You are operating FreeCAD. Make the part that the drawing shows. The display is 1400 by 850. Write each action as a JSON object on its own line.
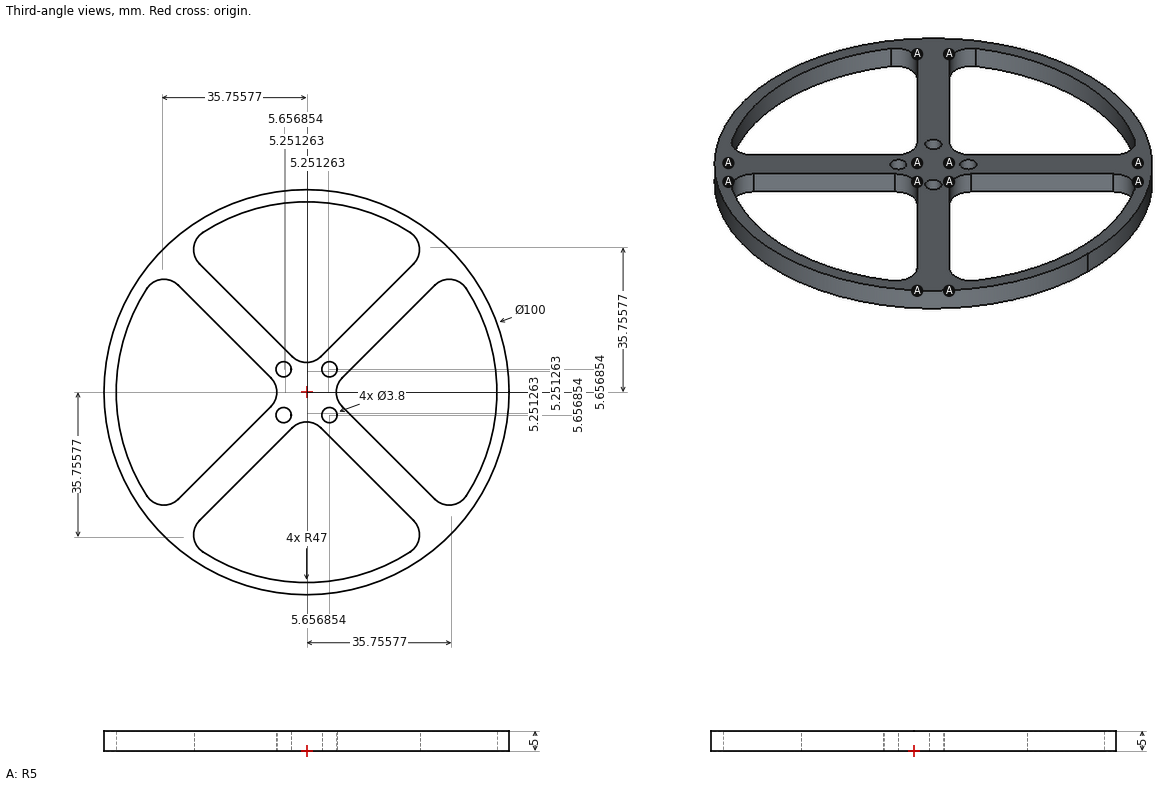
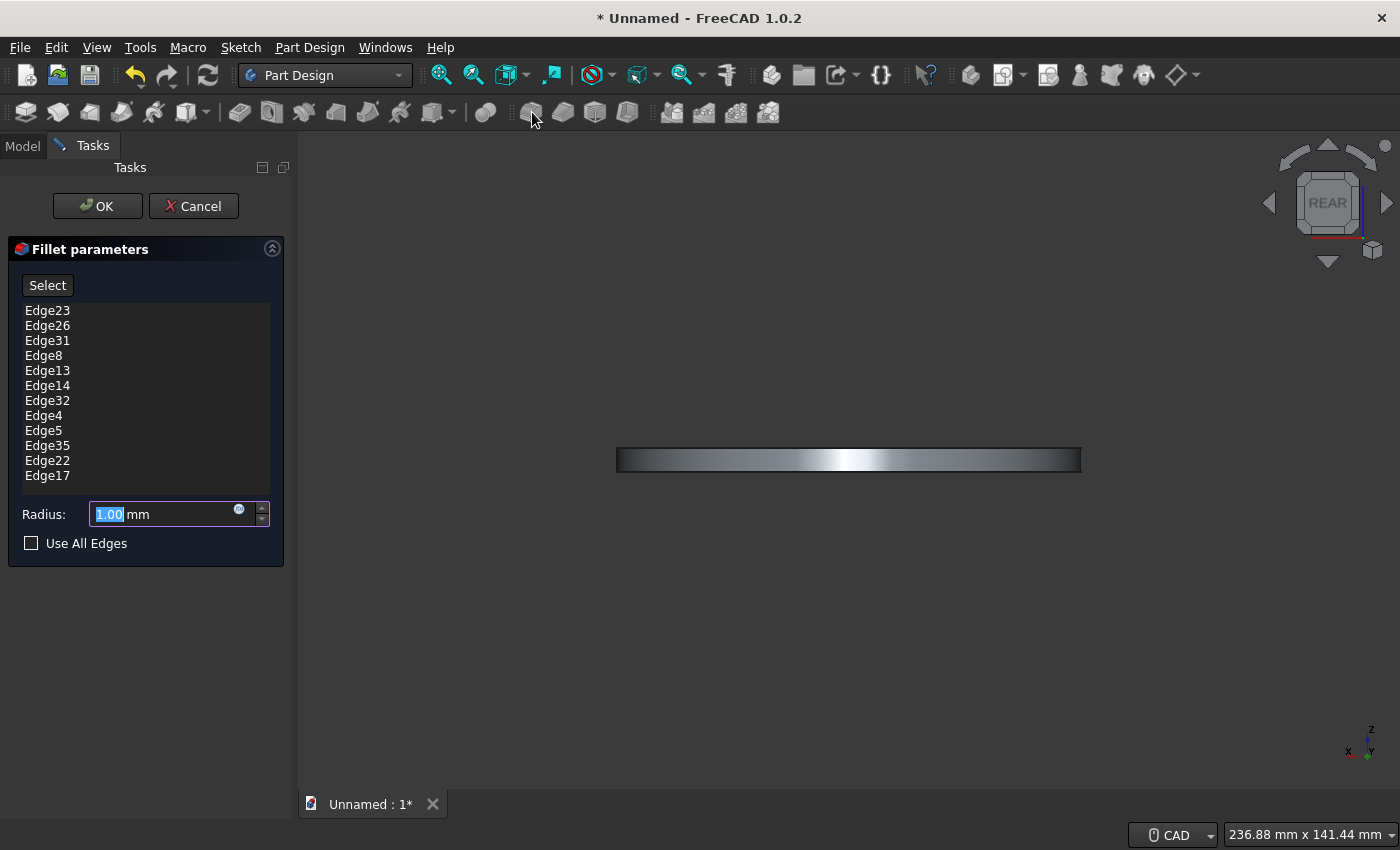
{"action": "type", "text": "5"}
{"action": "key", "text": "Tab"}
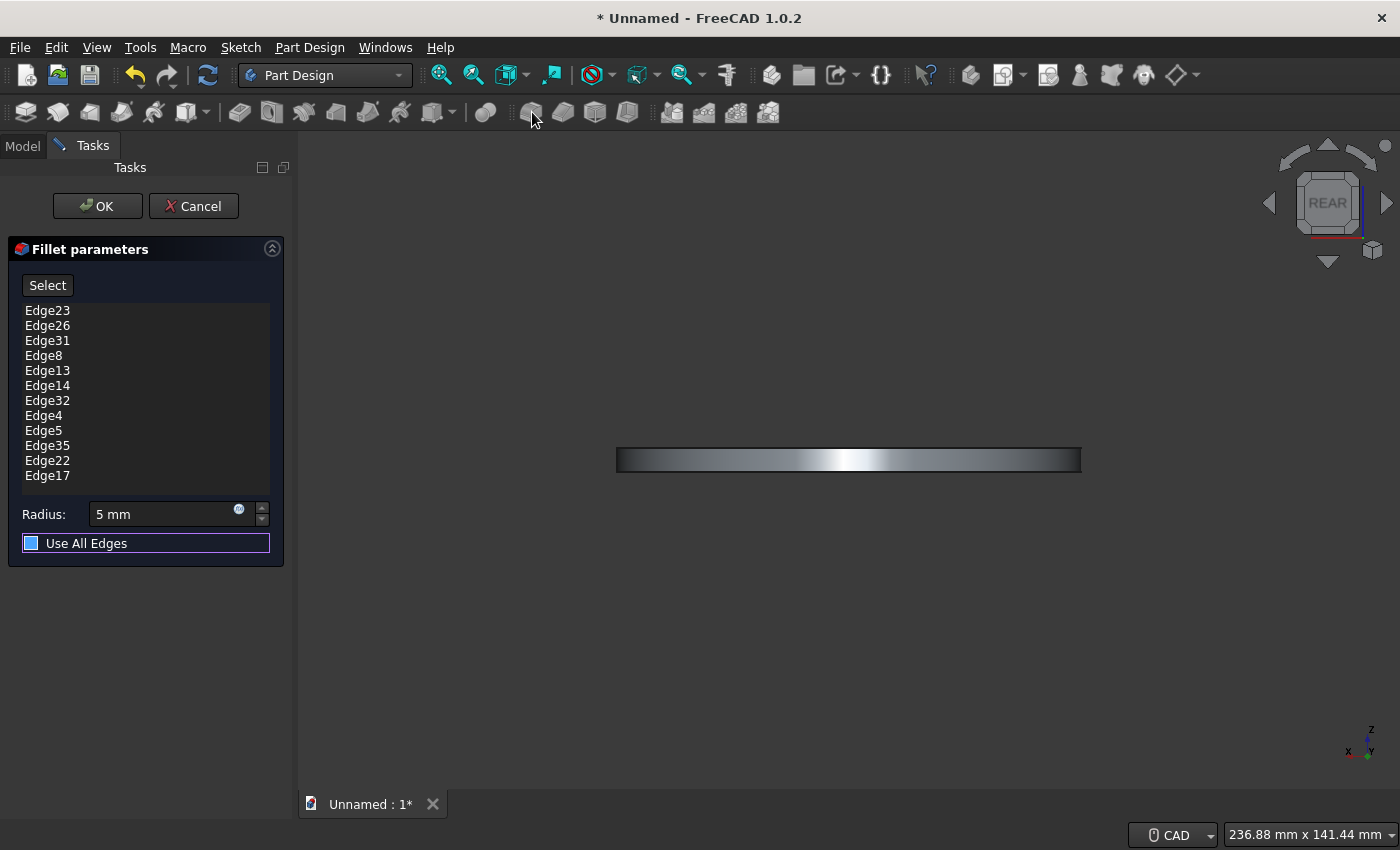
{"action": "left_click", "coordinate": [98, 206]}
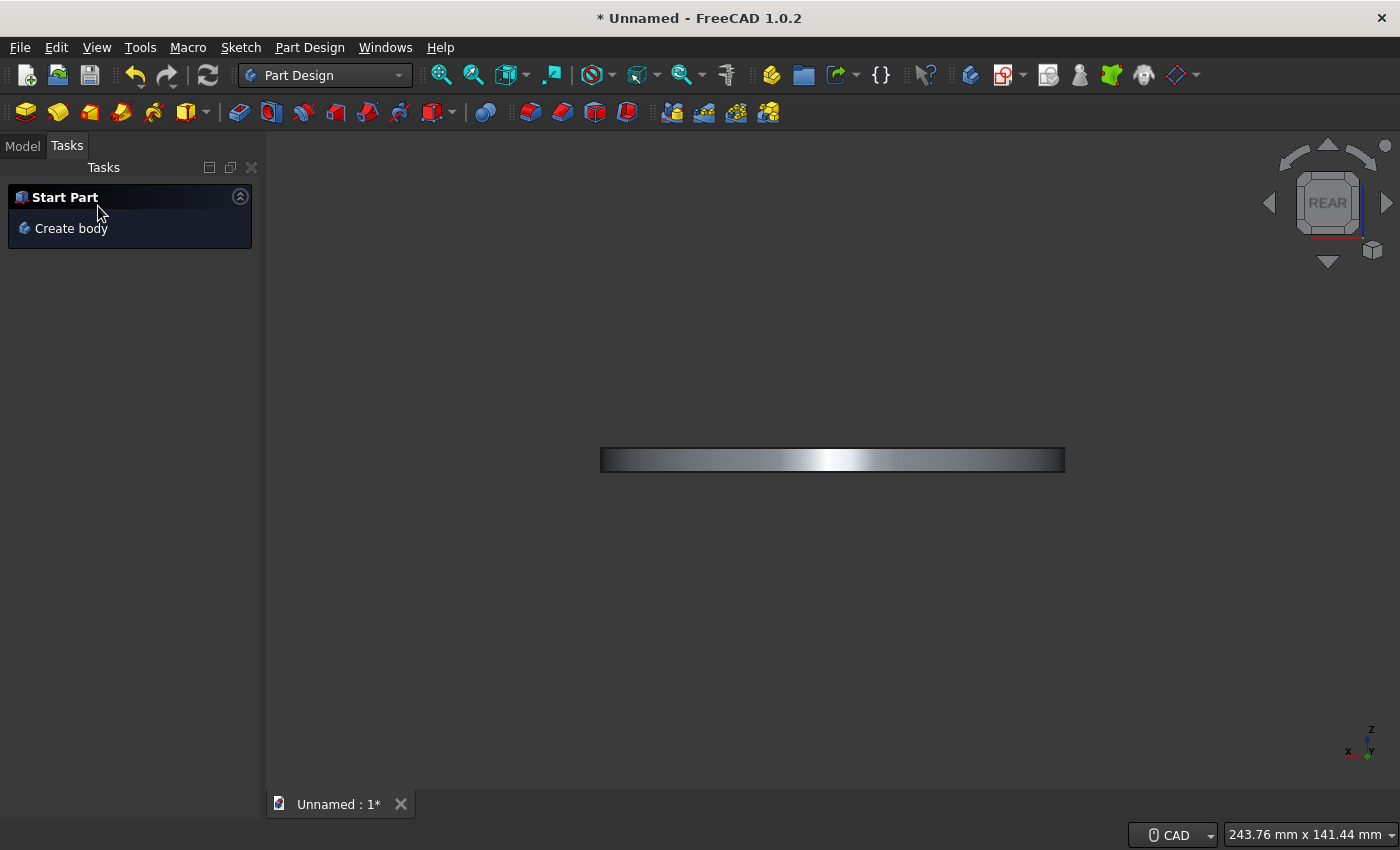
{"action": "left_click", "coordinate": [442, 76]}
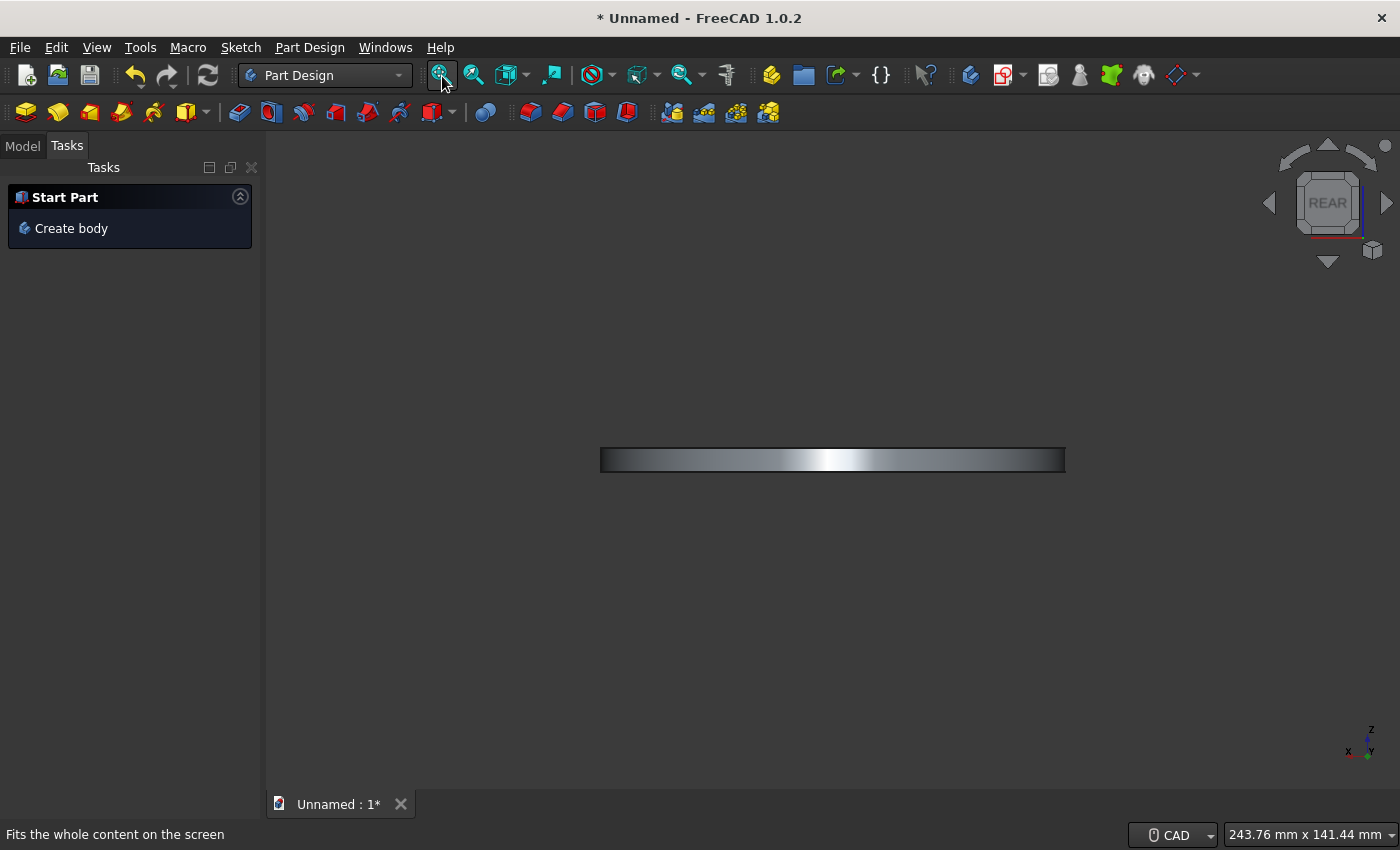
{"action": "key", "text": "0"}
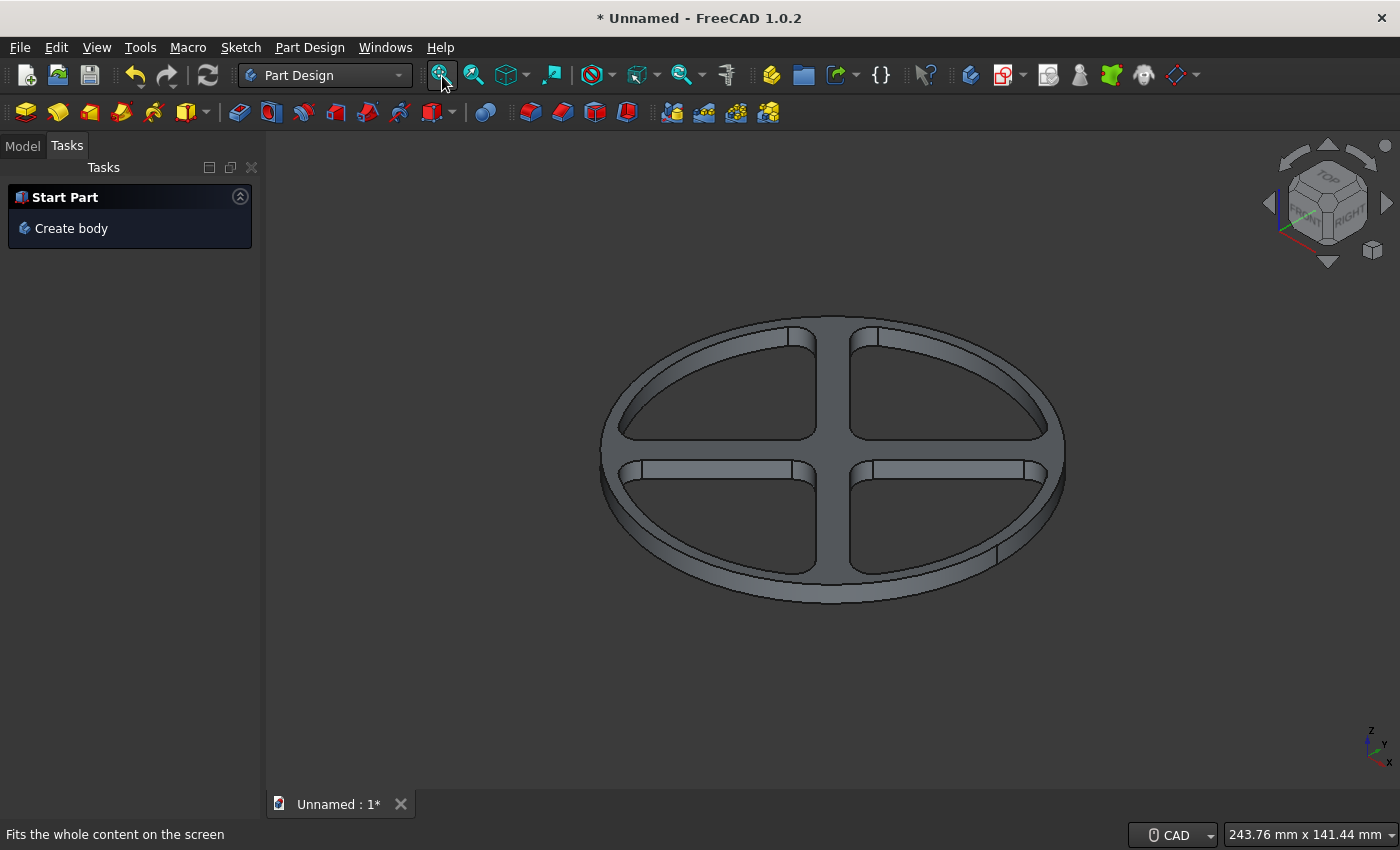
{"action": "left_click", "coordinate": [833, 449]}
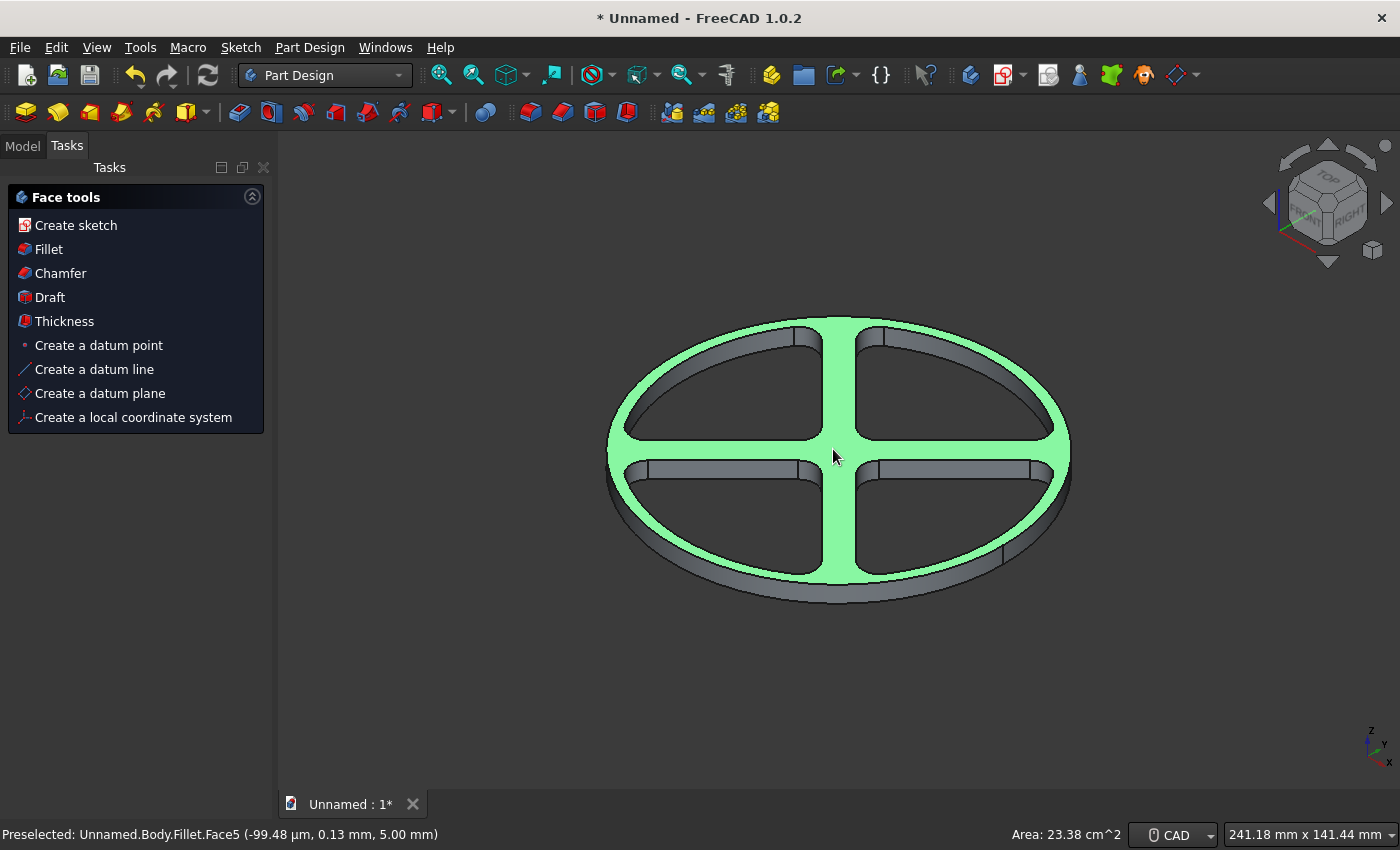
{"action": "left_click", "coordinate": [1004, 76]}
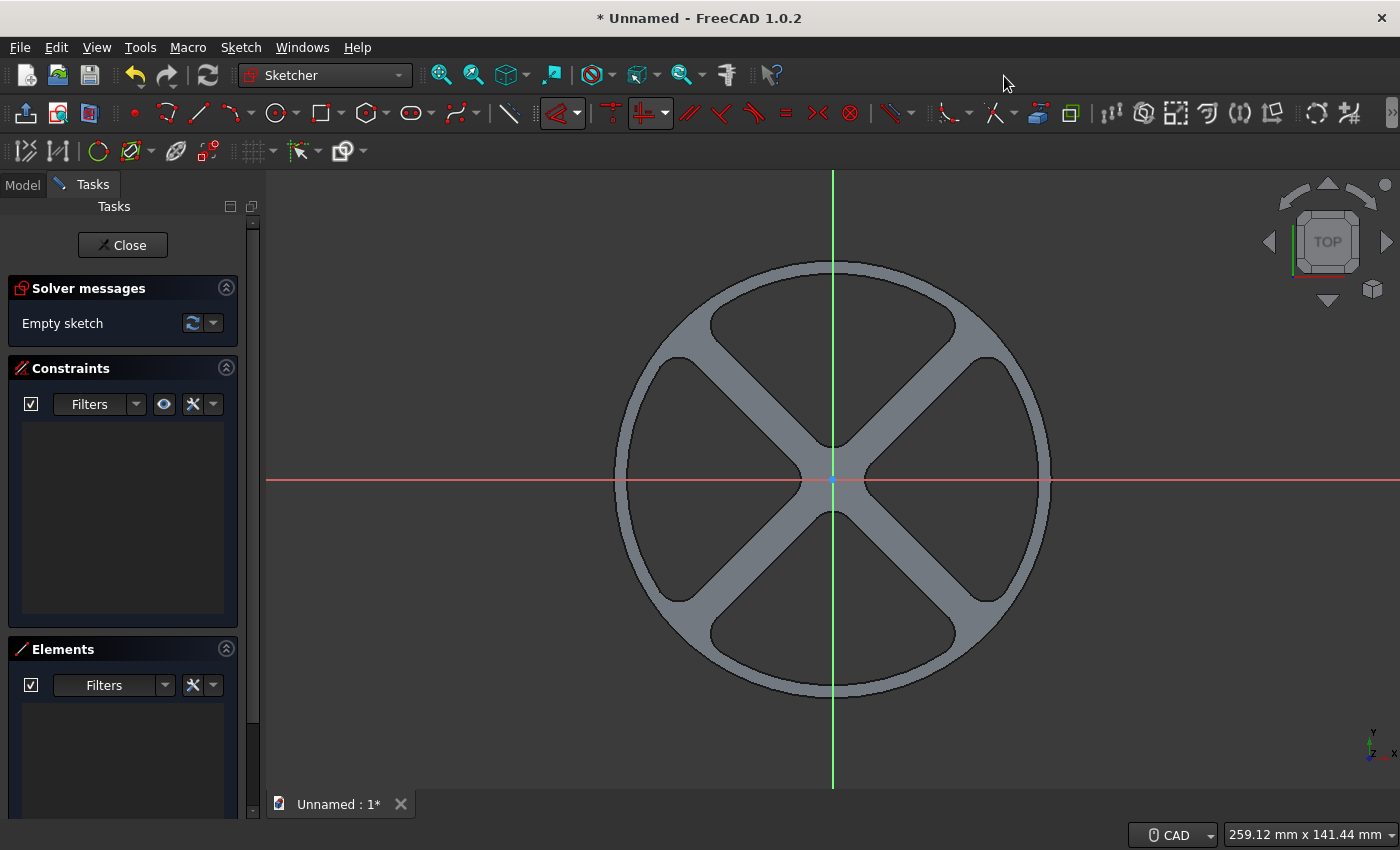
{"action": "scroll", "coordinate": [846, 480], "scroll_direction": "up", "scroll_amount": 9}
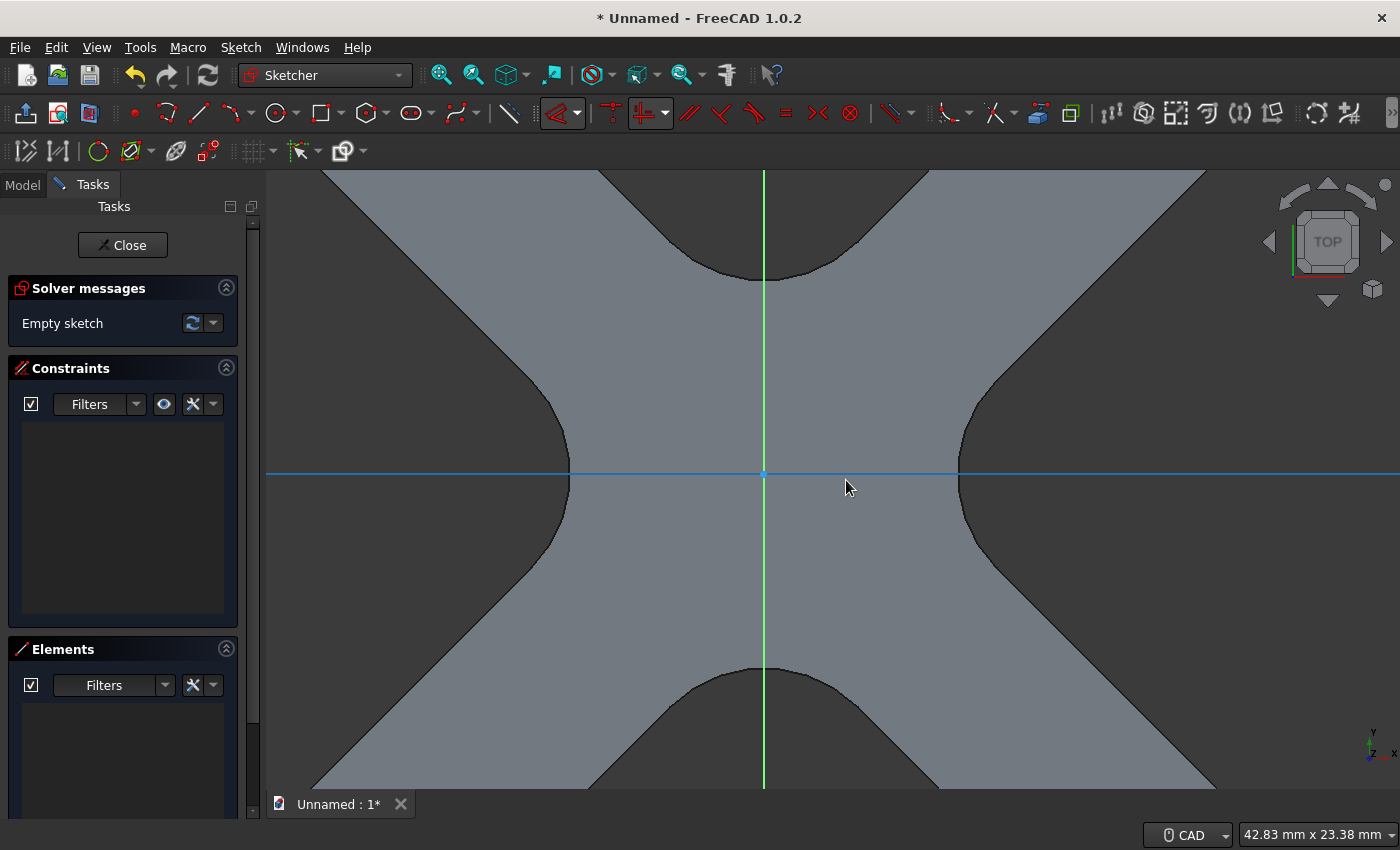
{"action": "left_click", "coordinate": [276, 114]}